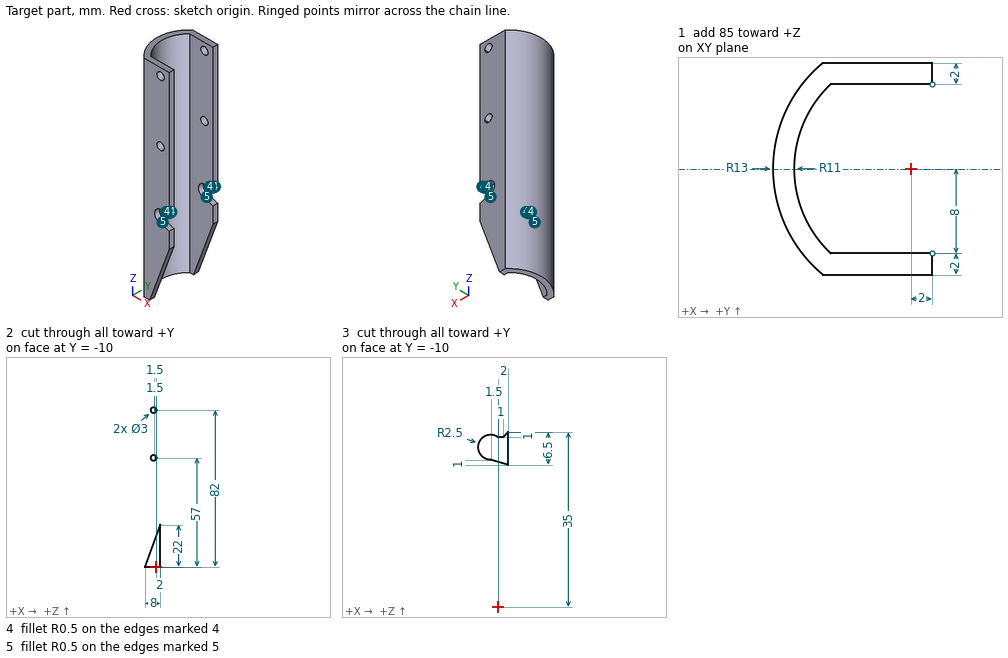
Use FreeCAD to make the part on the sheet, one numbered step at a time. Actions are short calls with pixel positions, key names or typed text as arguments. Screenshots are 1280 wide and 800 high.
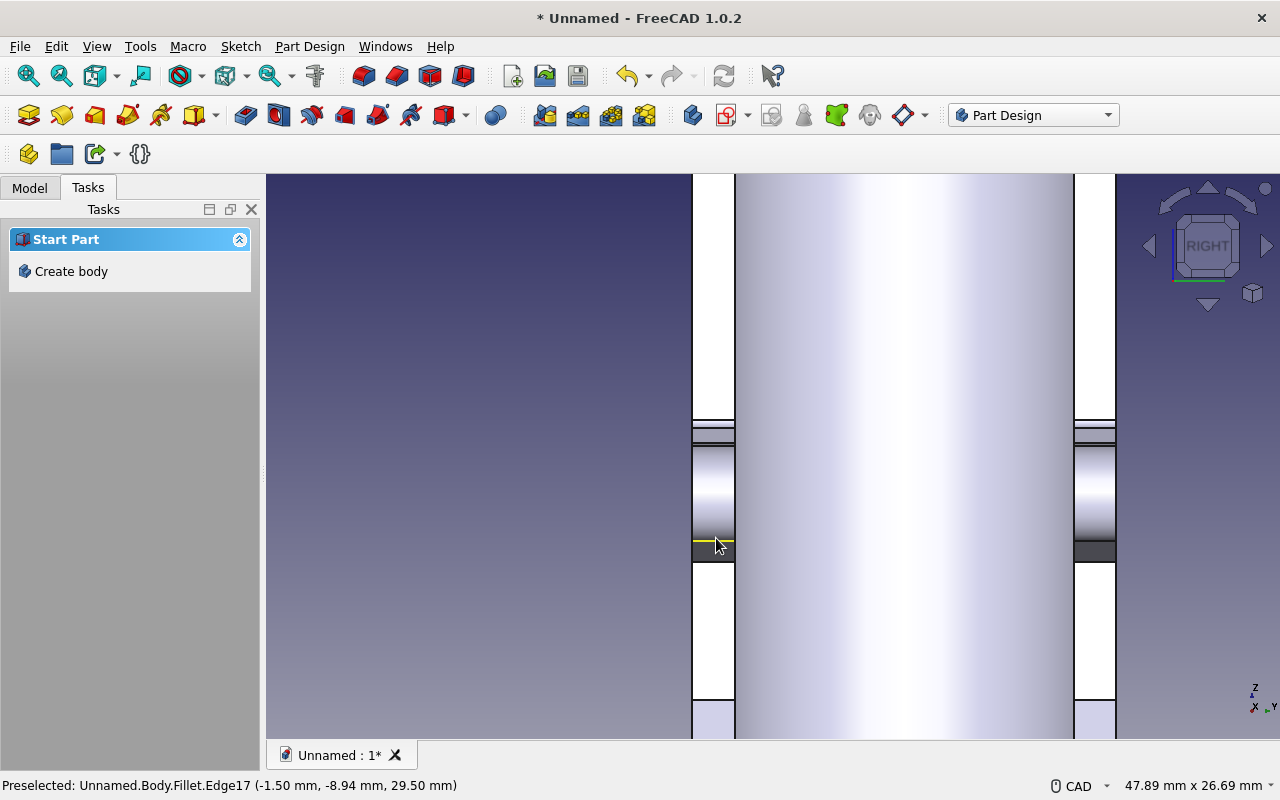
click(29, 76)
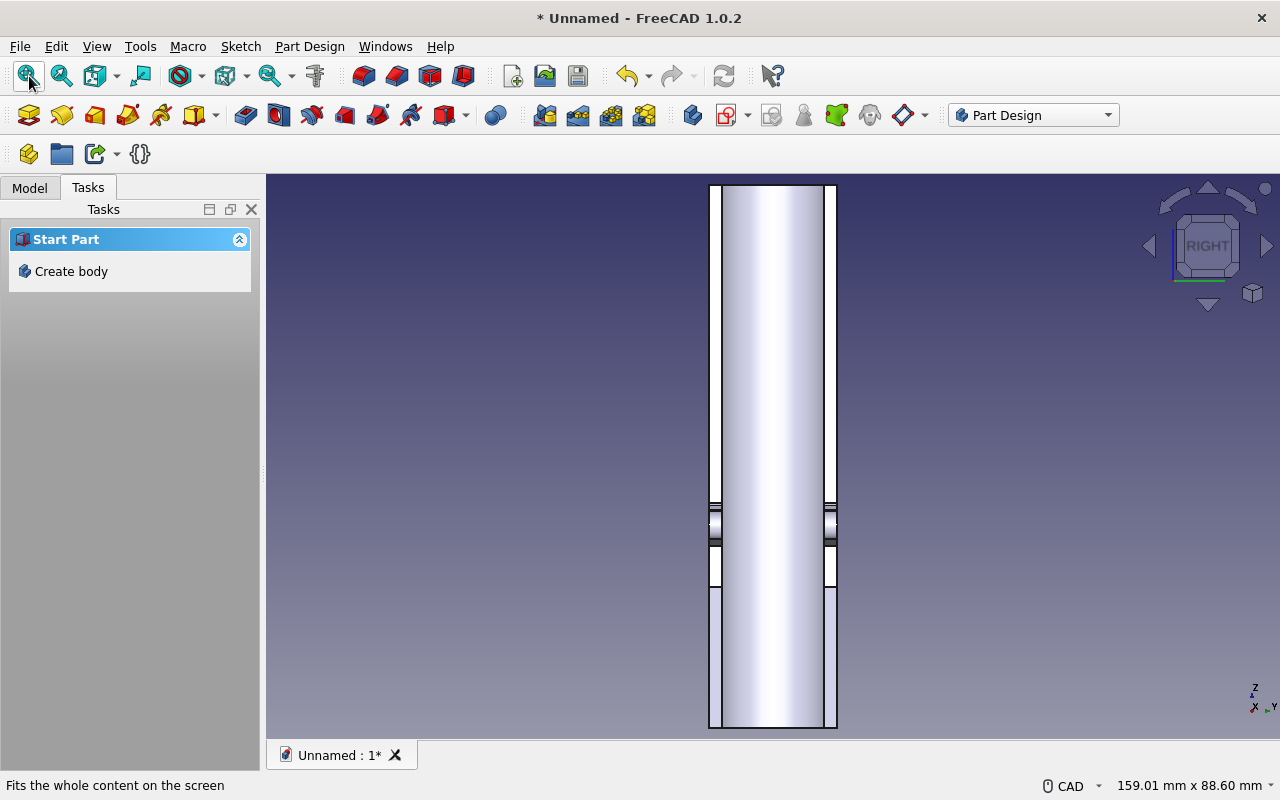
key(5)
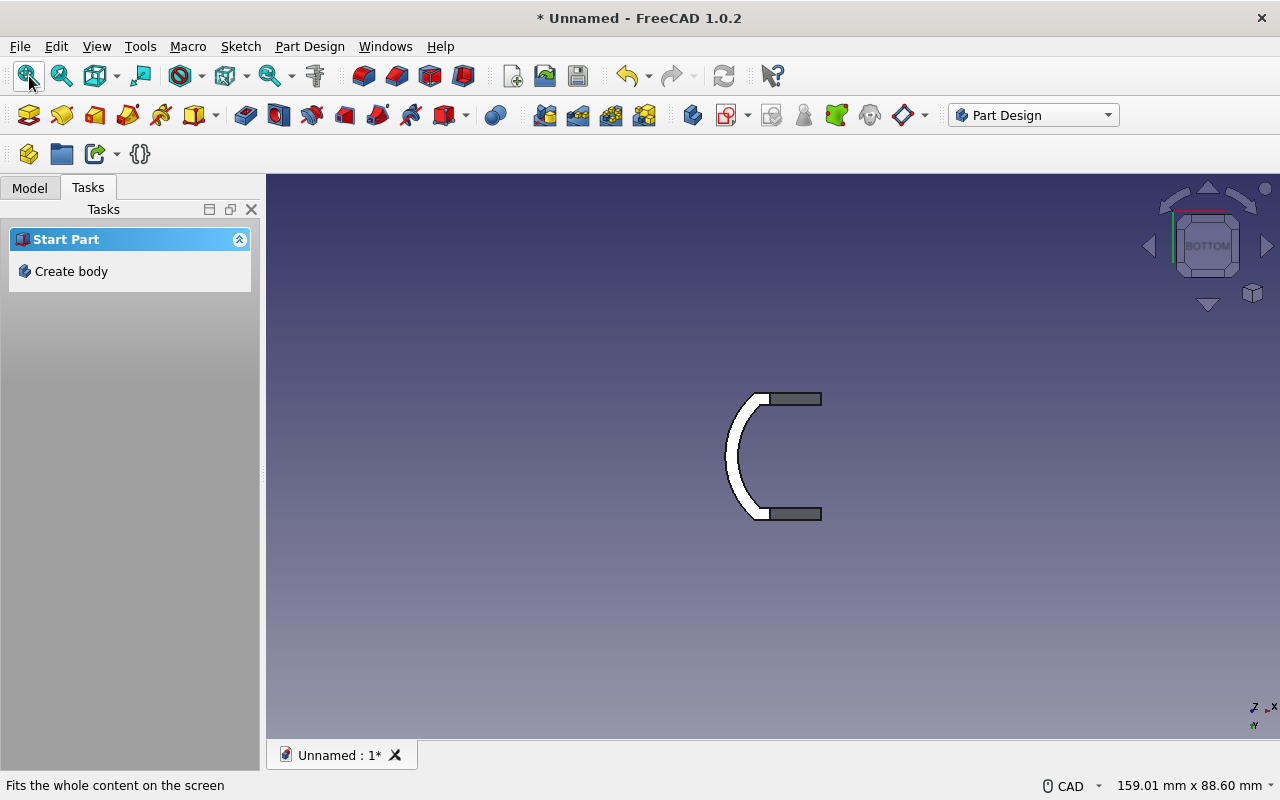
key(v)
key(f)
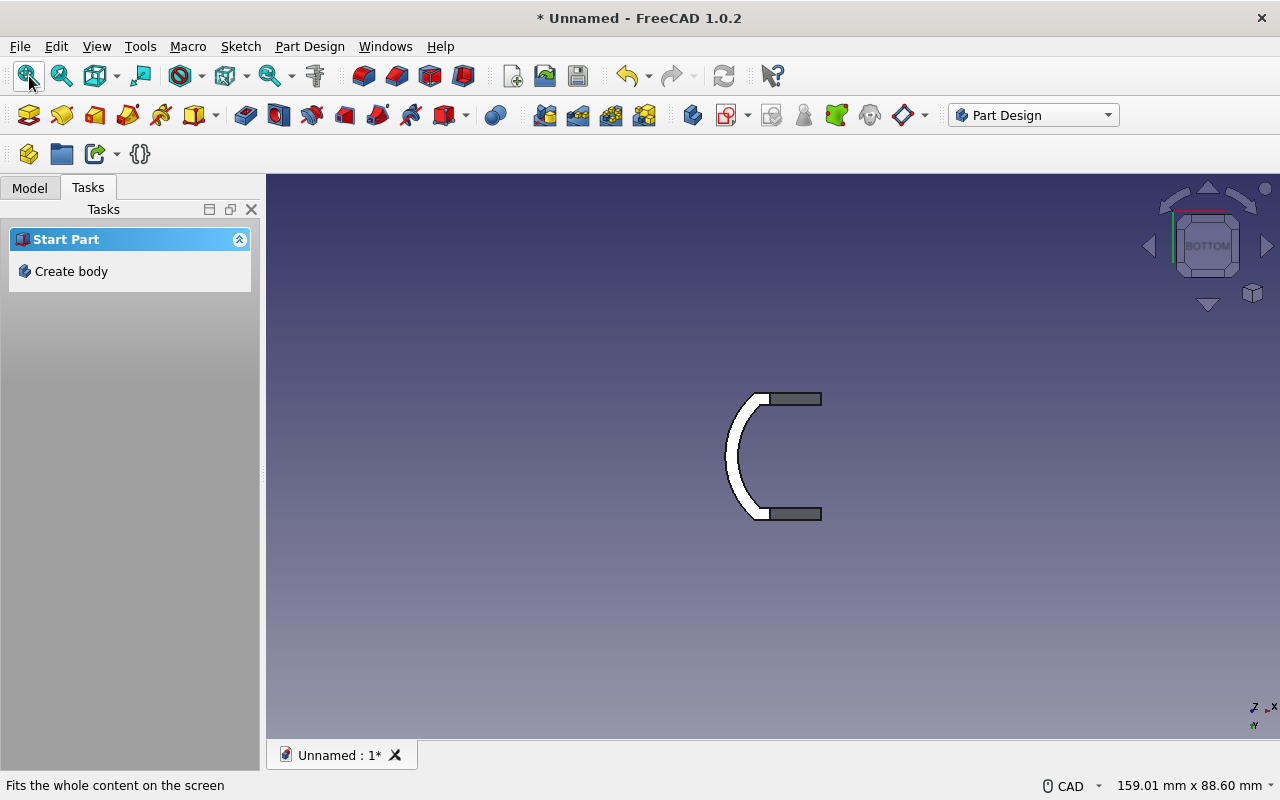
scroll(799, 398, up, 6)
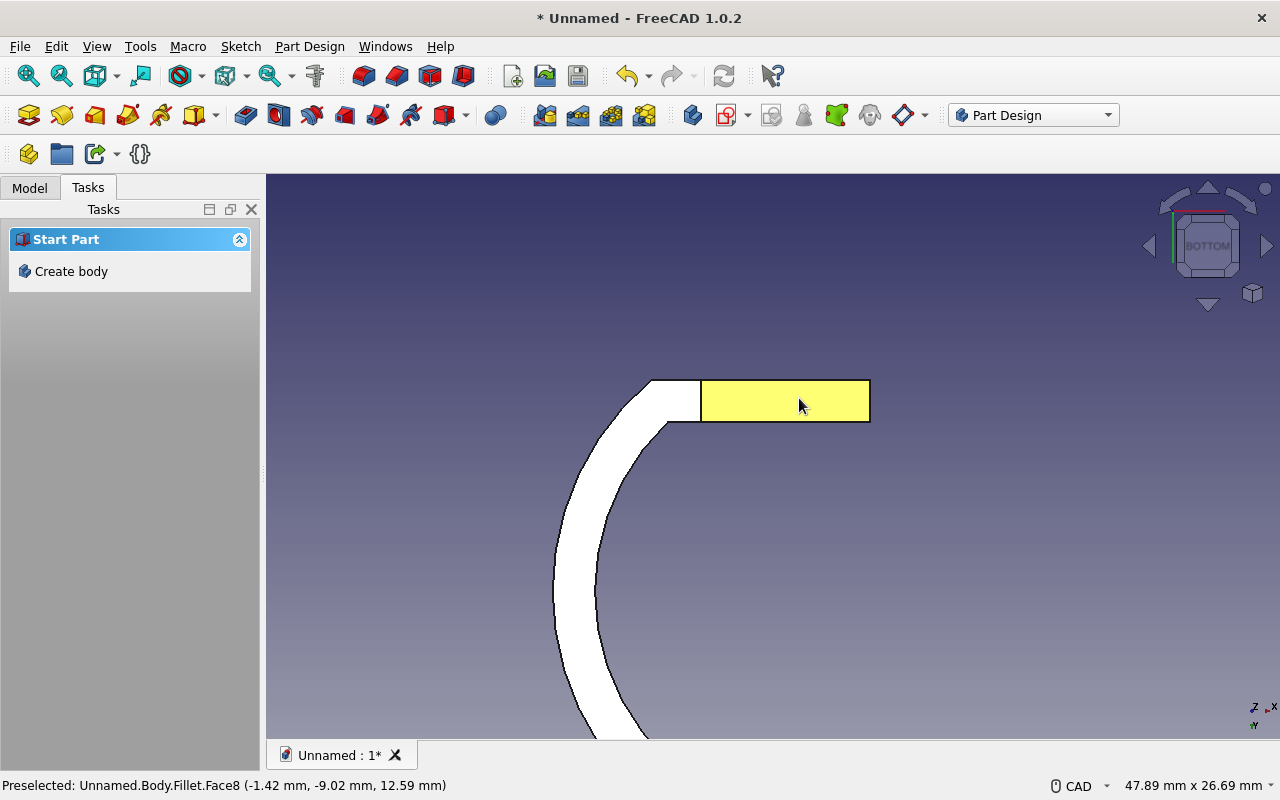
key(v)
key(f)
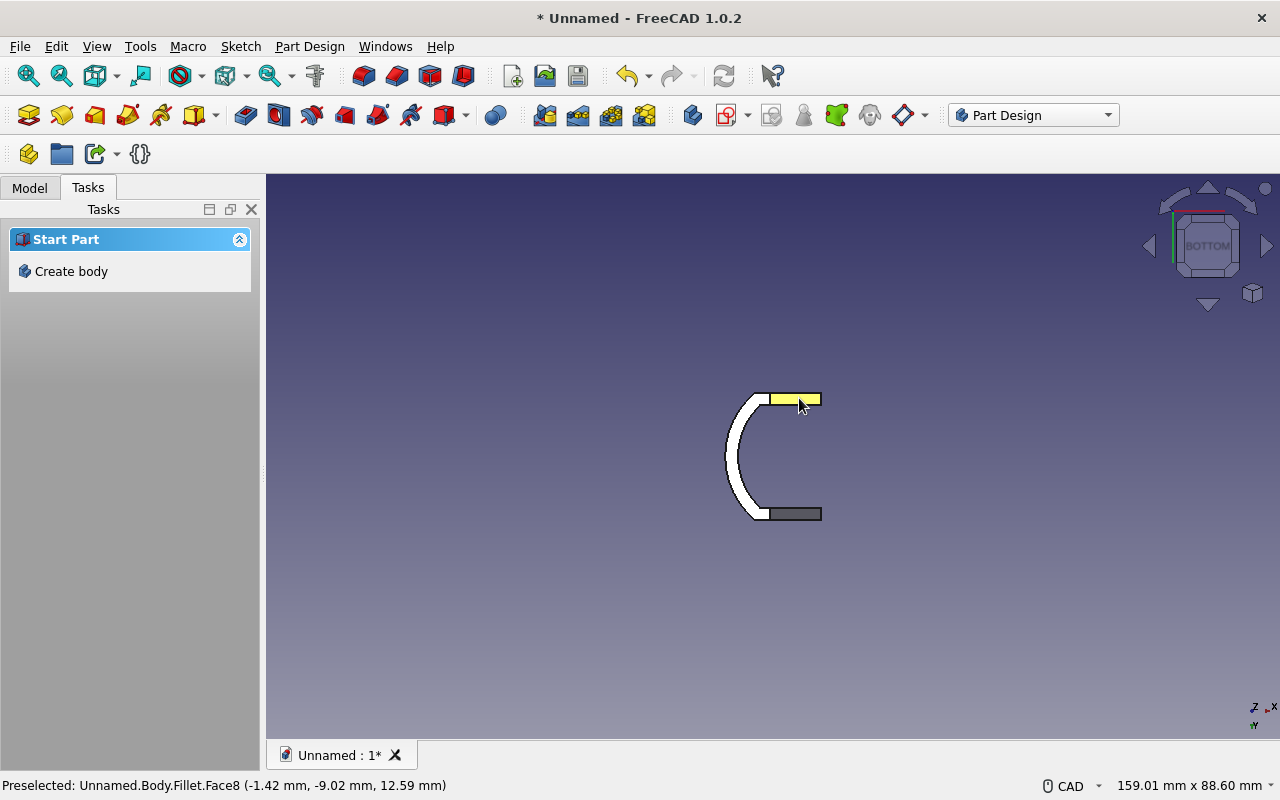
key(4)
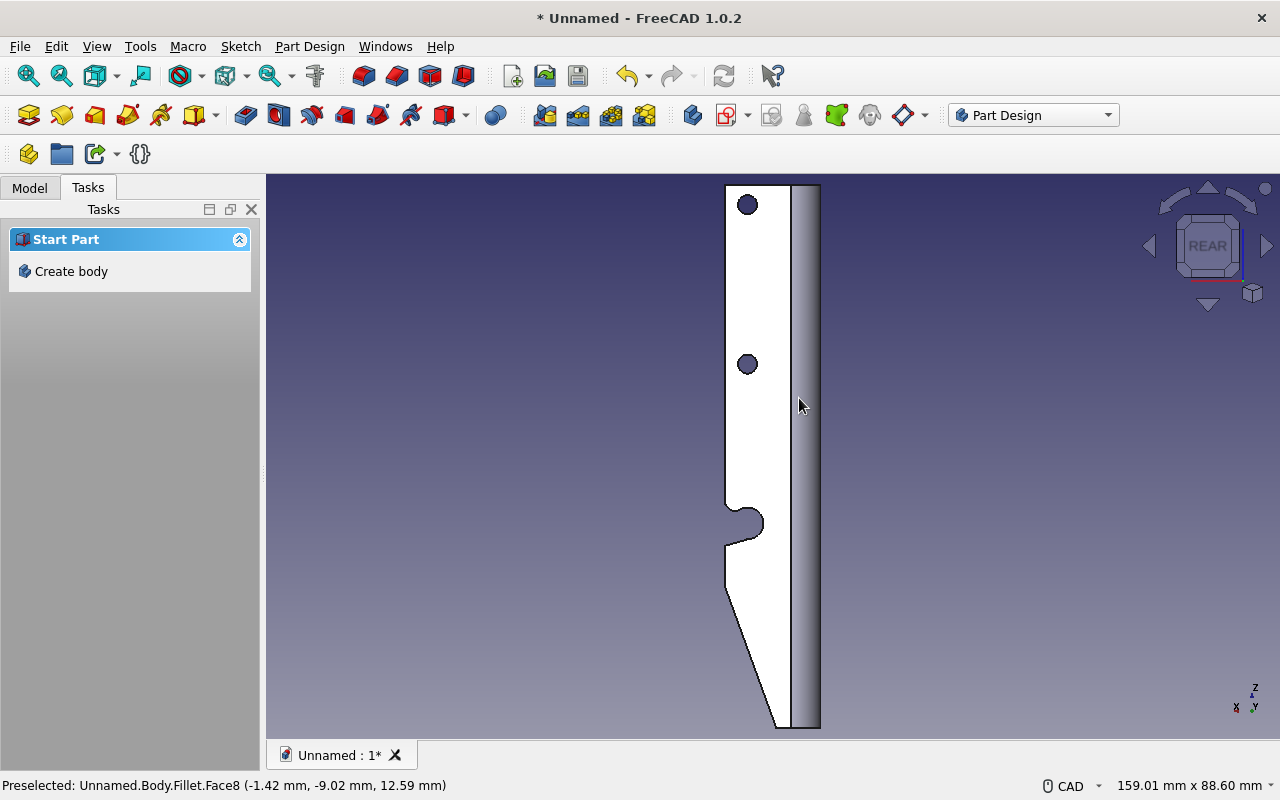
scroll(747, 538, up, 6)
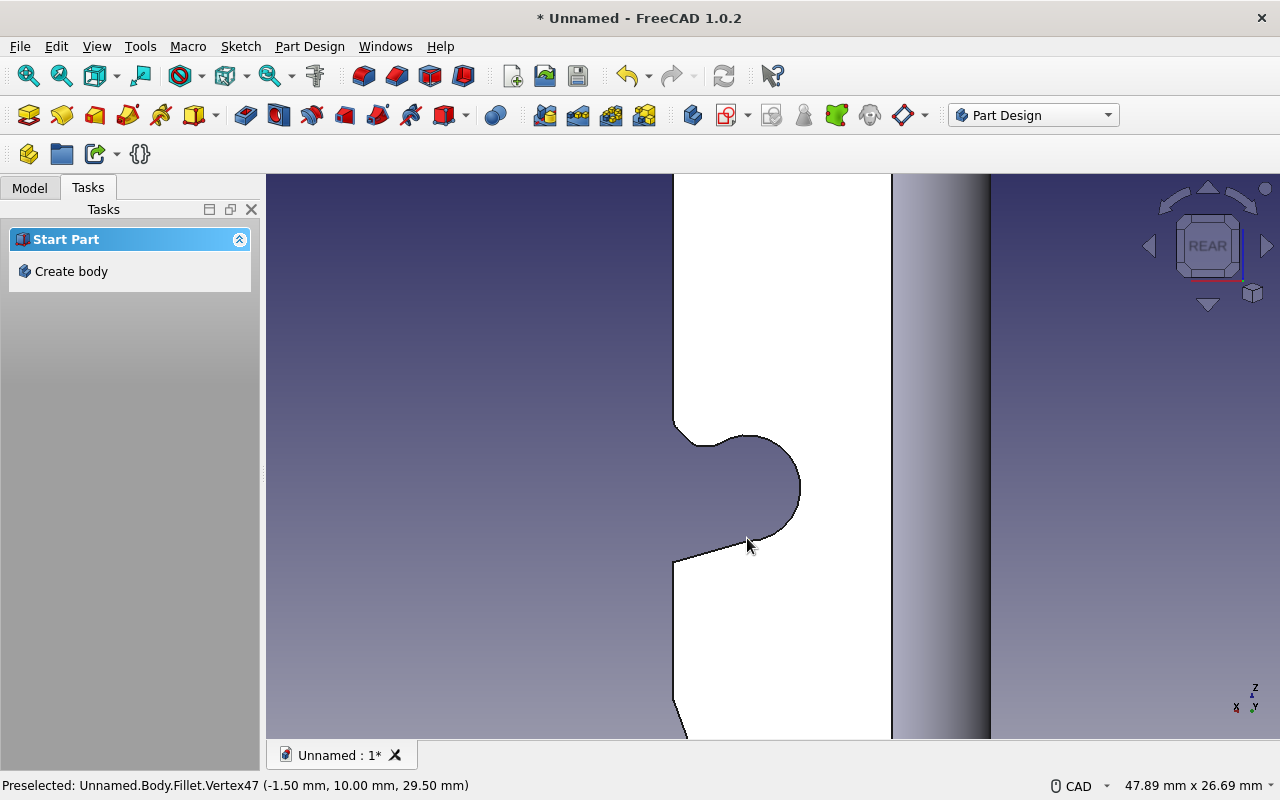
click(29, 76)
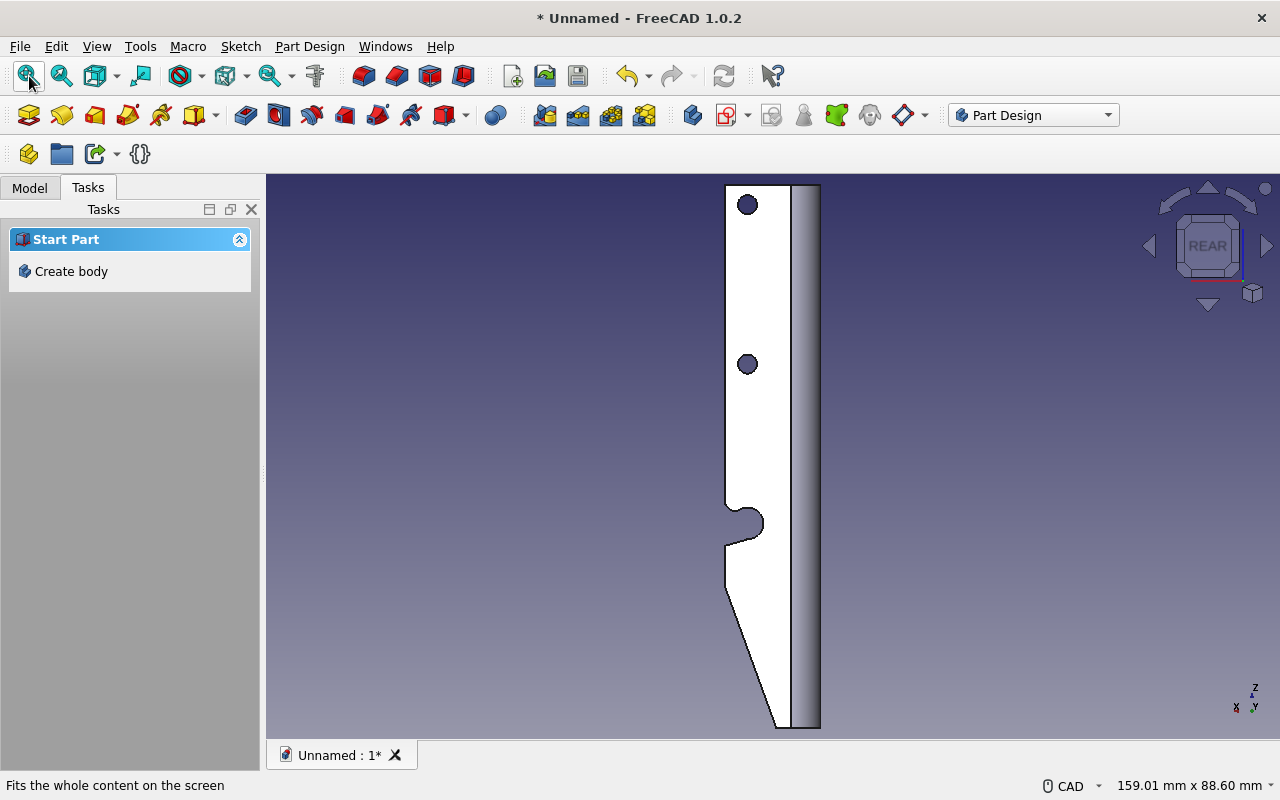
key(6)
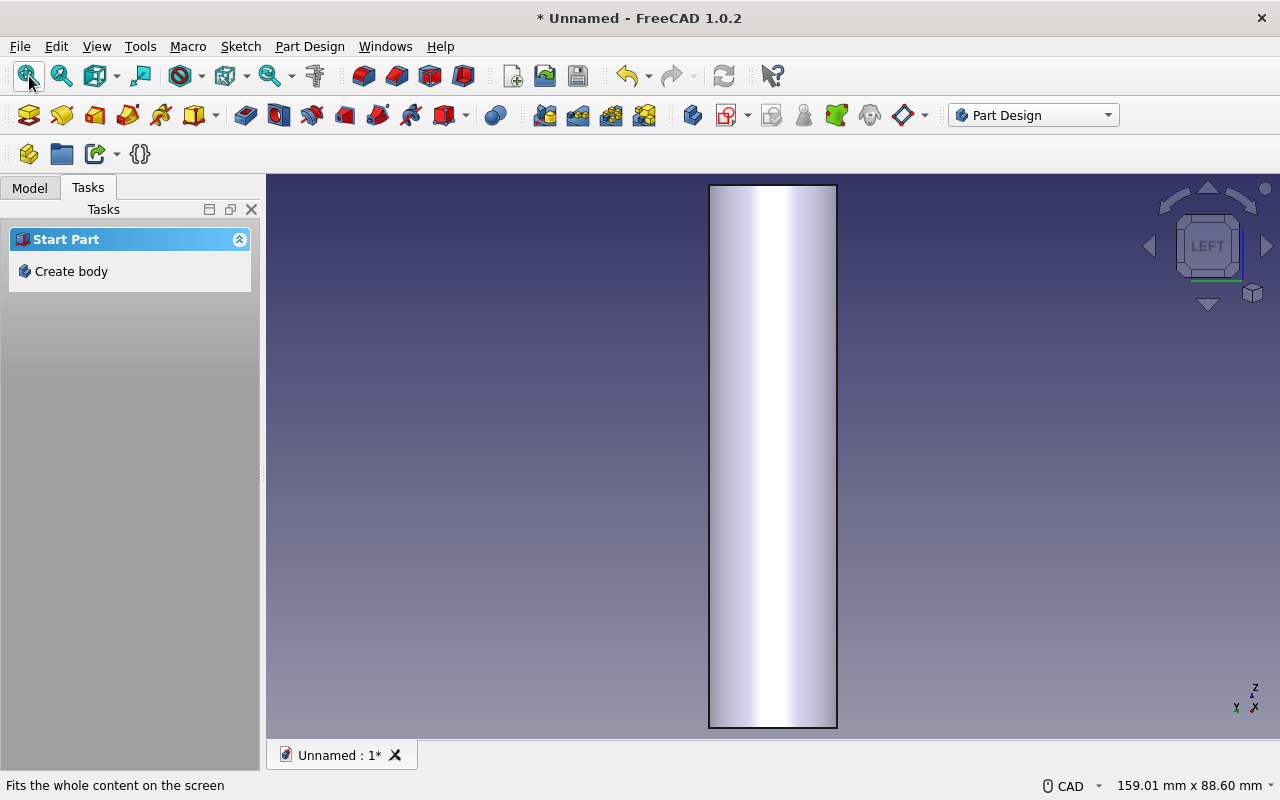
scroll(830, 538, up, 6)